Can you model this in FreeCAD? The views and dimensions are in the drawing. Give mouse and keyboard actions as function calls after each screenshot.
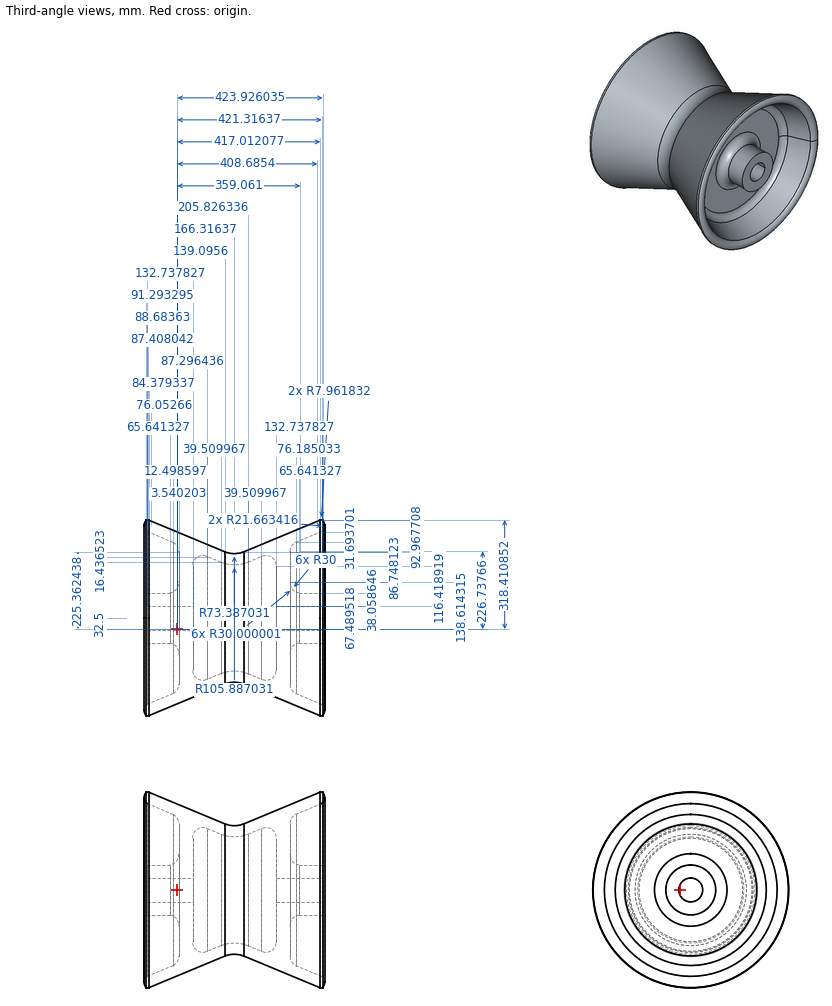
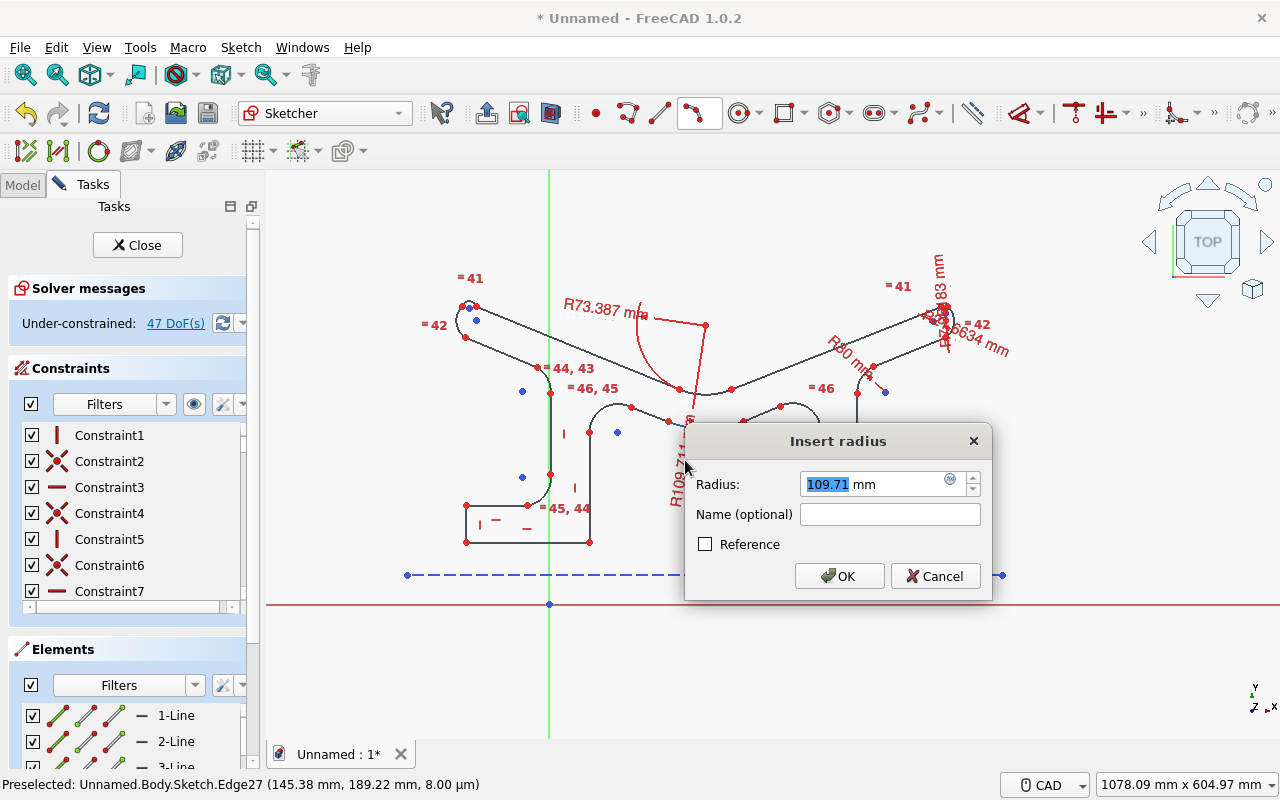
text(105.887031)
key(Return)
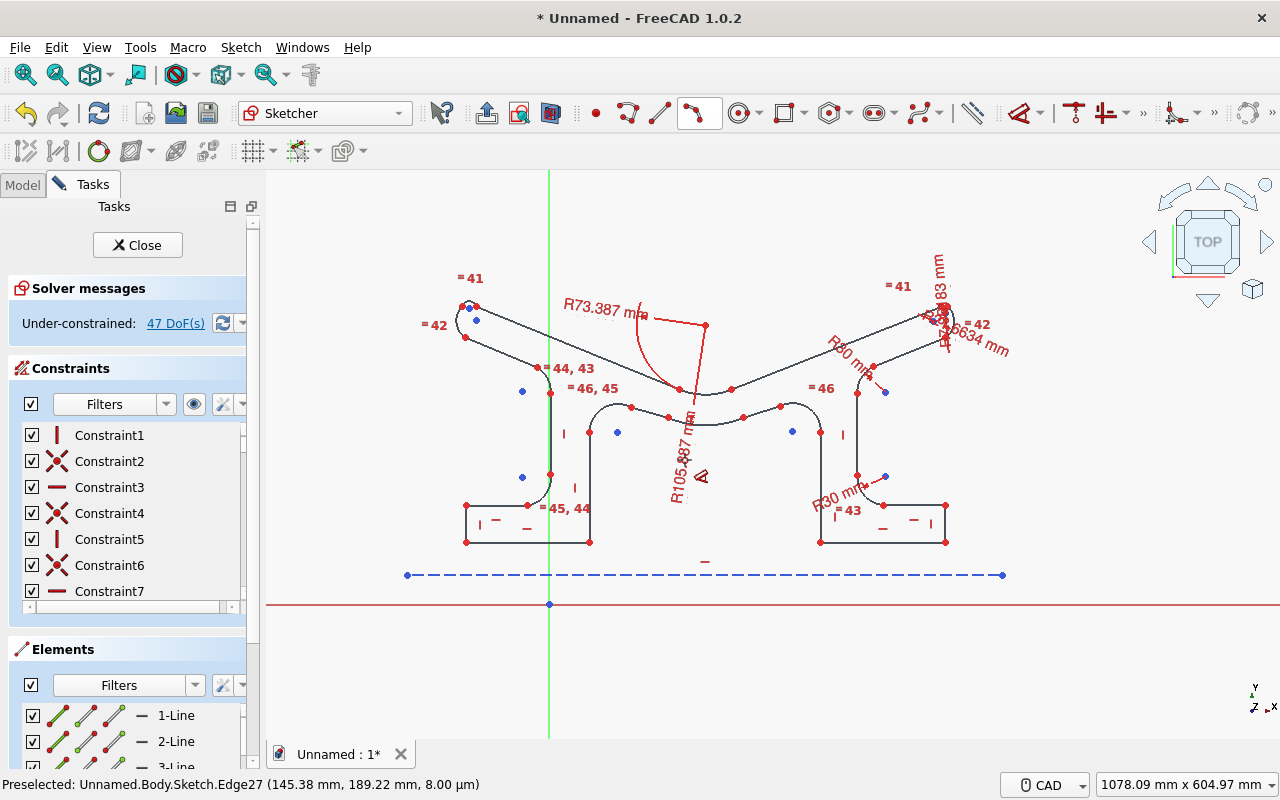
scroll(408, 575, up, 2)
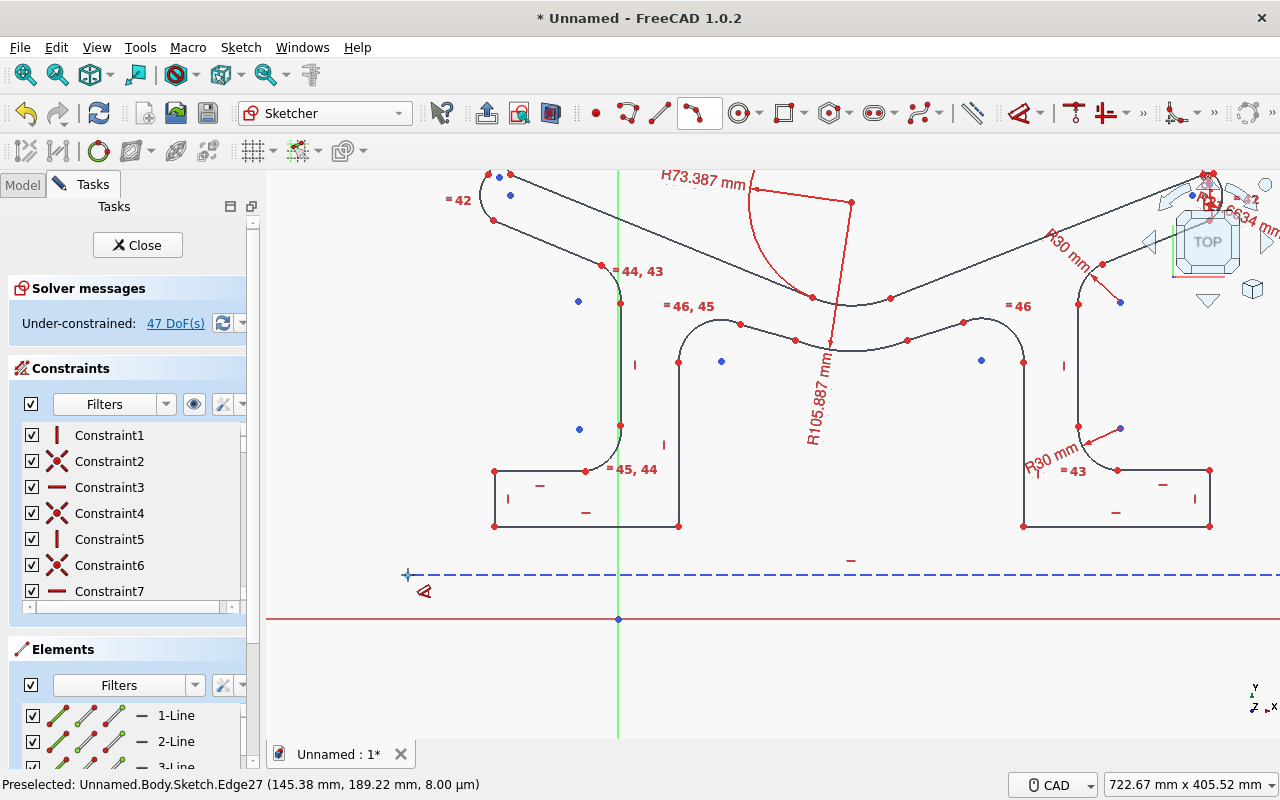
click(408, 575)
click(374, 597)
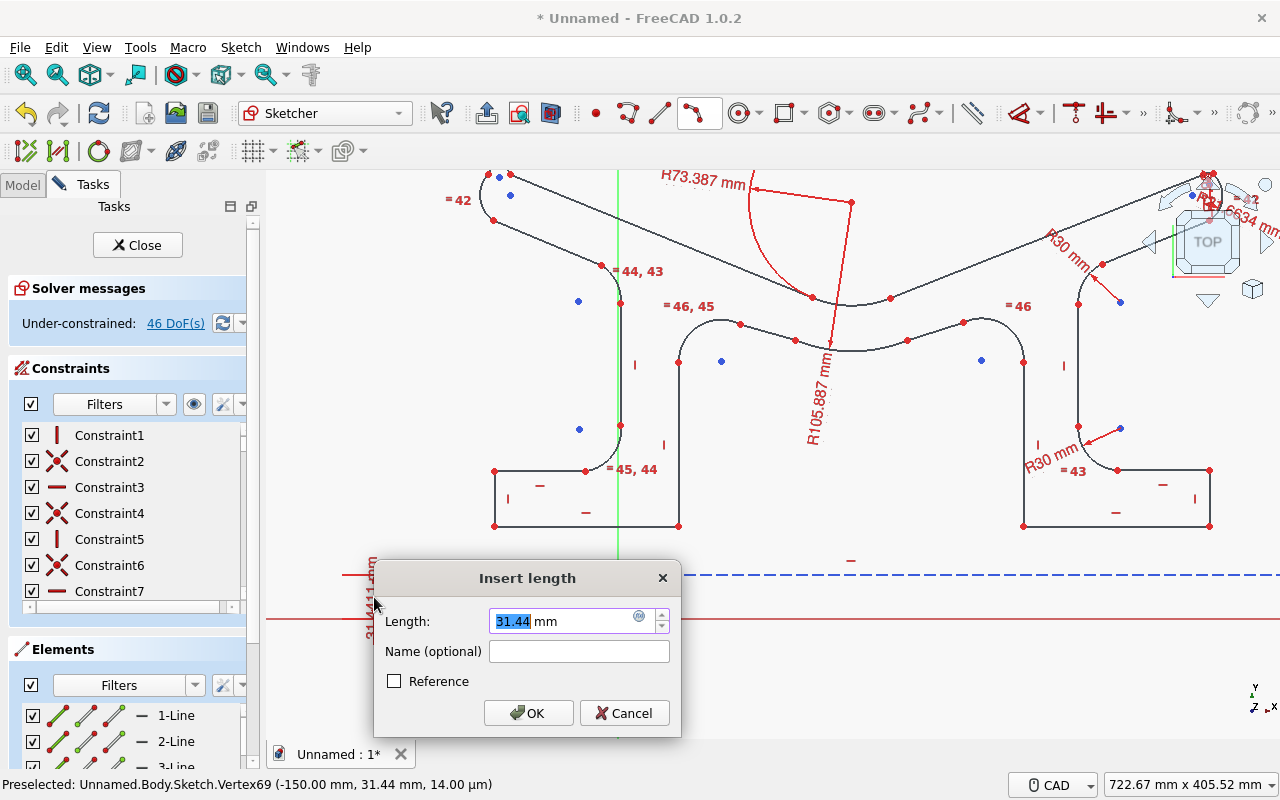
text(32.5)
key(Return)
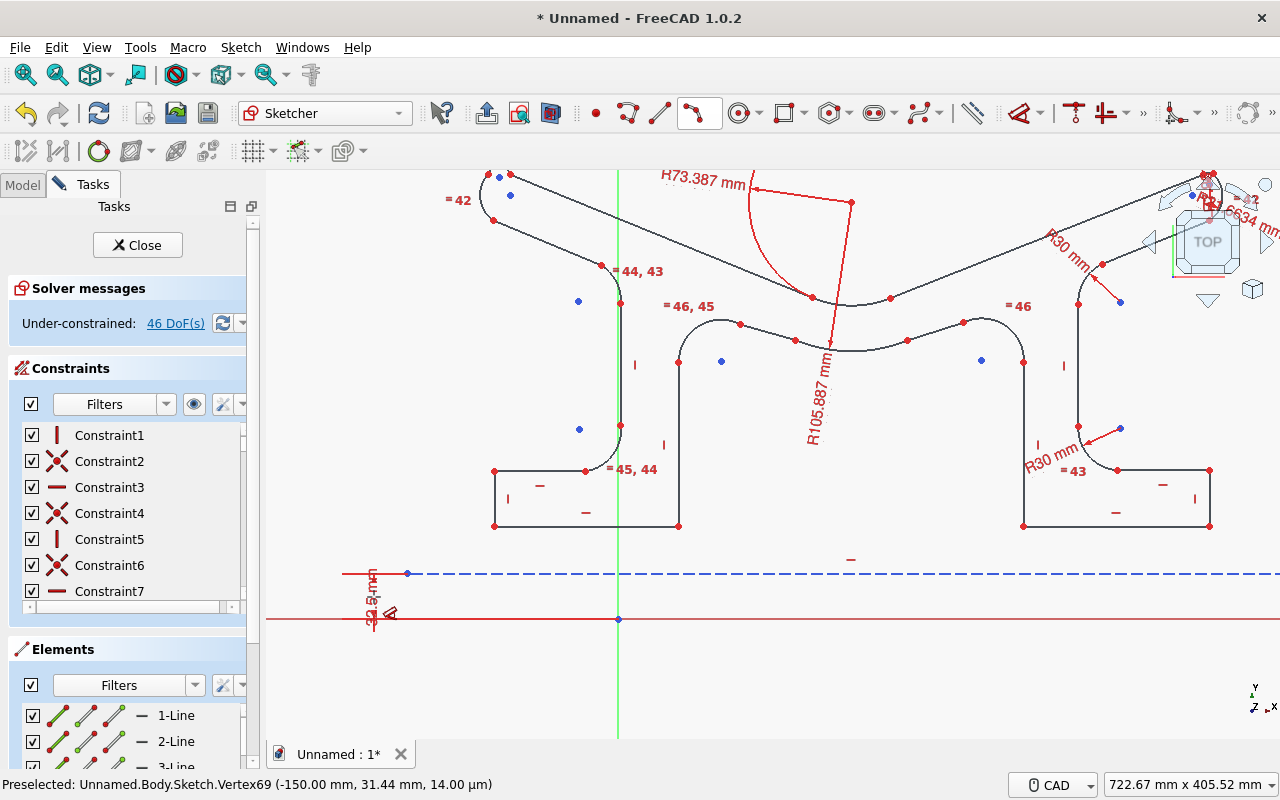
scroll(405, 575, down, 2)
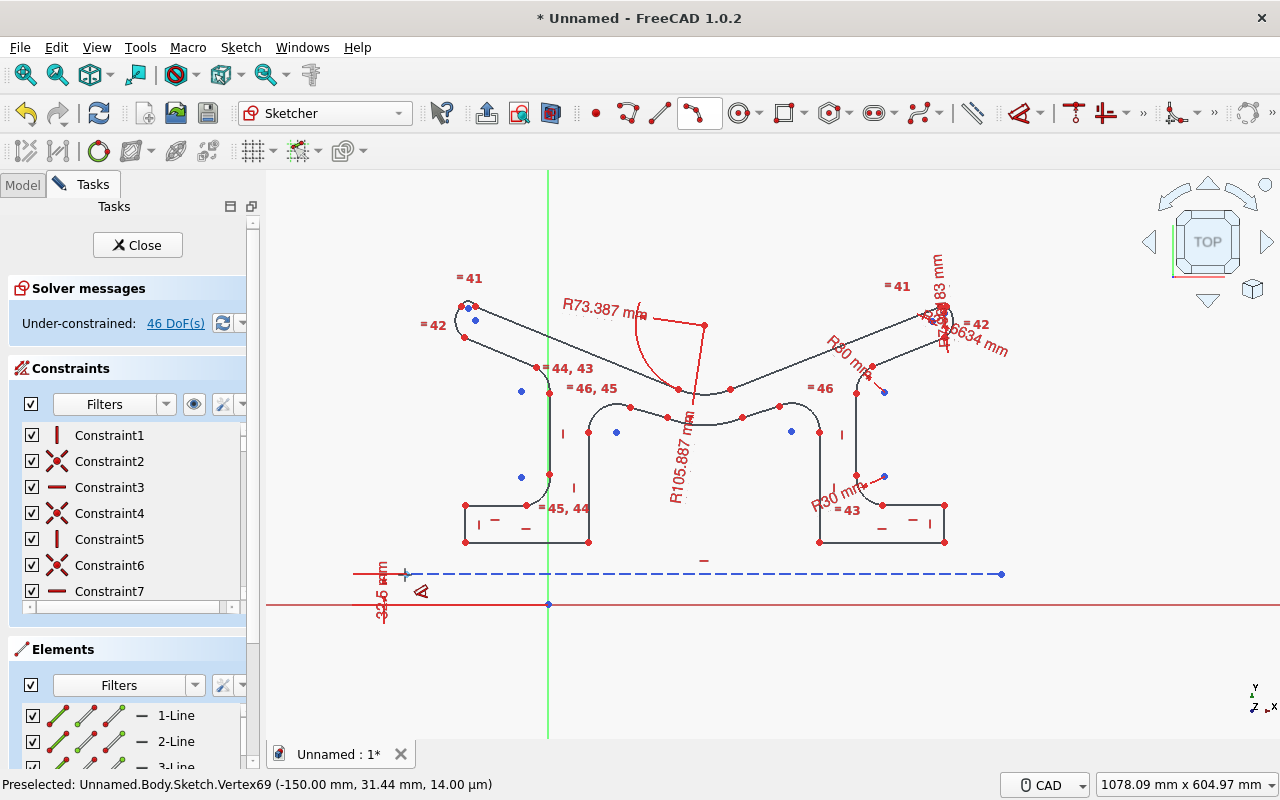
click(885, 392)
click(716, 639)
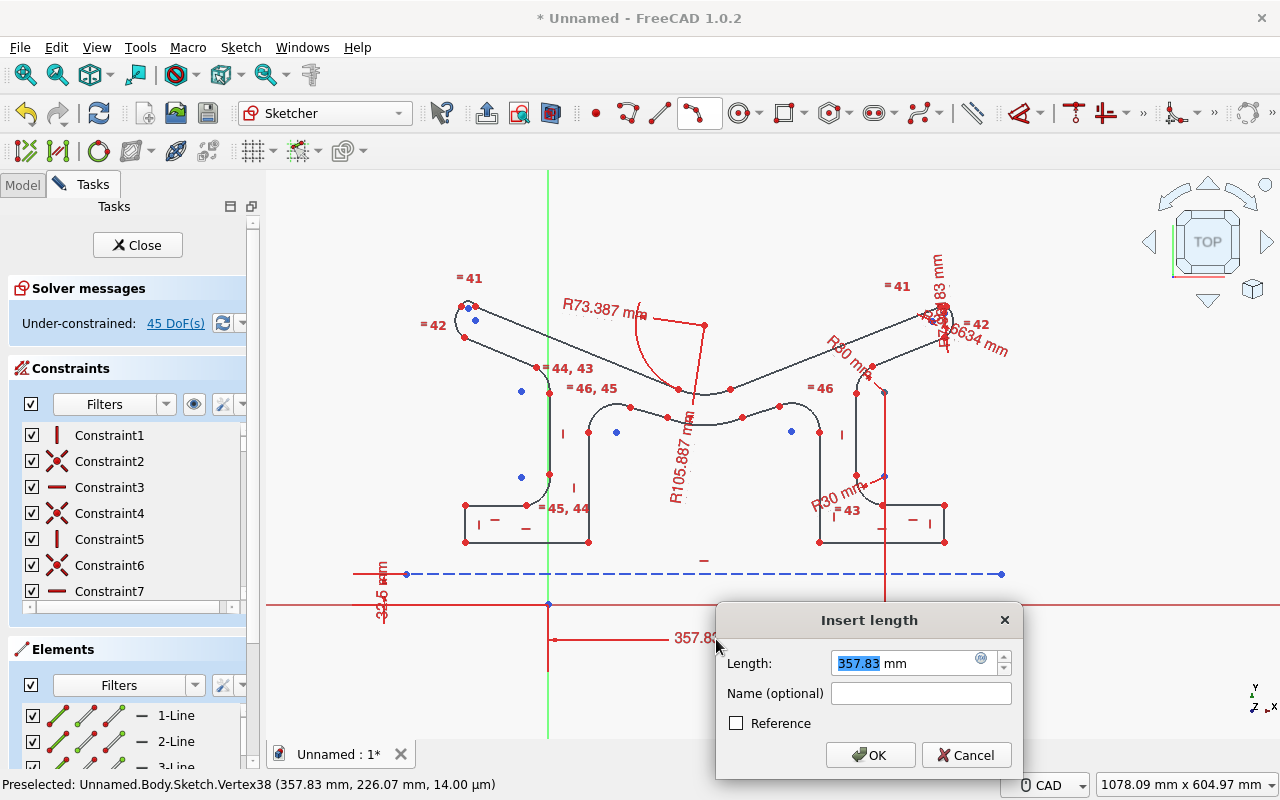
text(359.061)
key(Return)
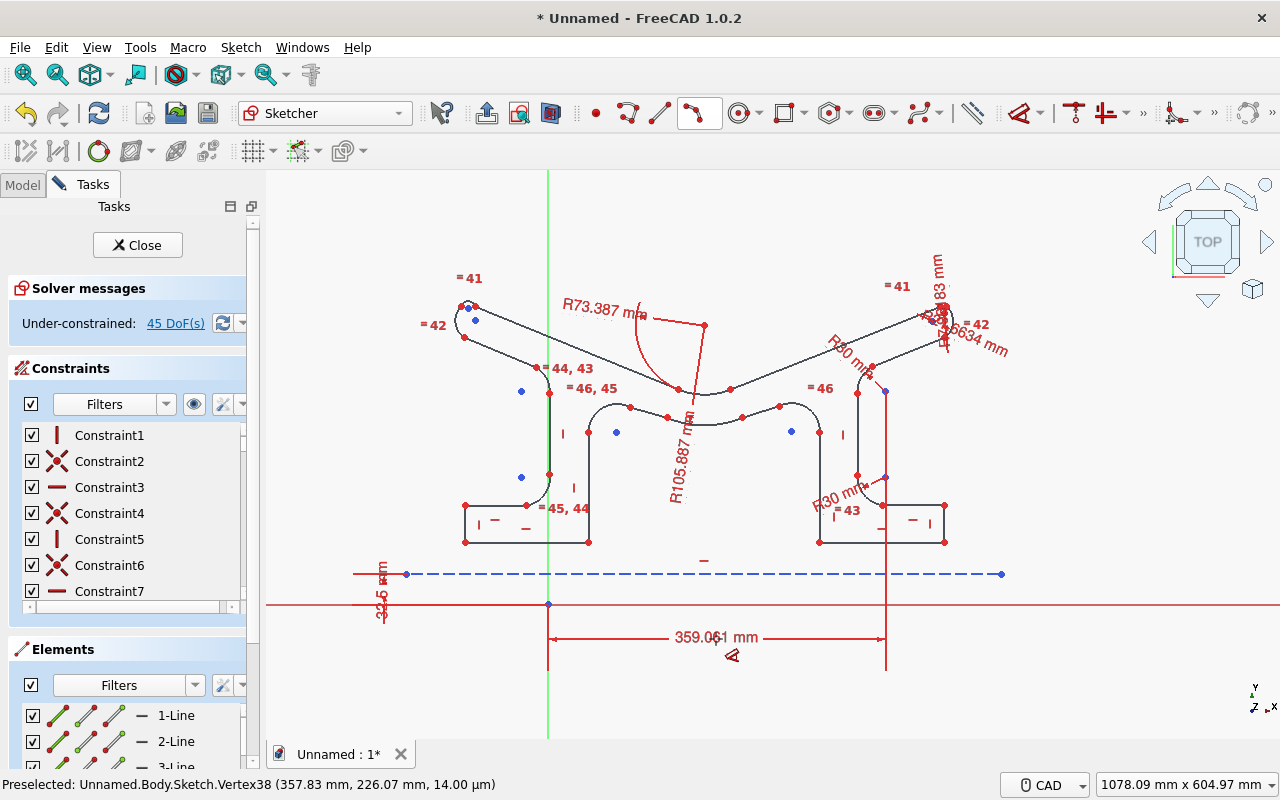
click(944, 532)
click(978, 524)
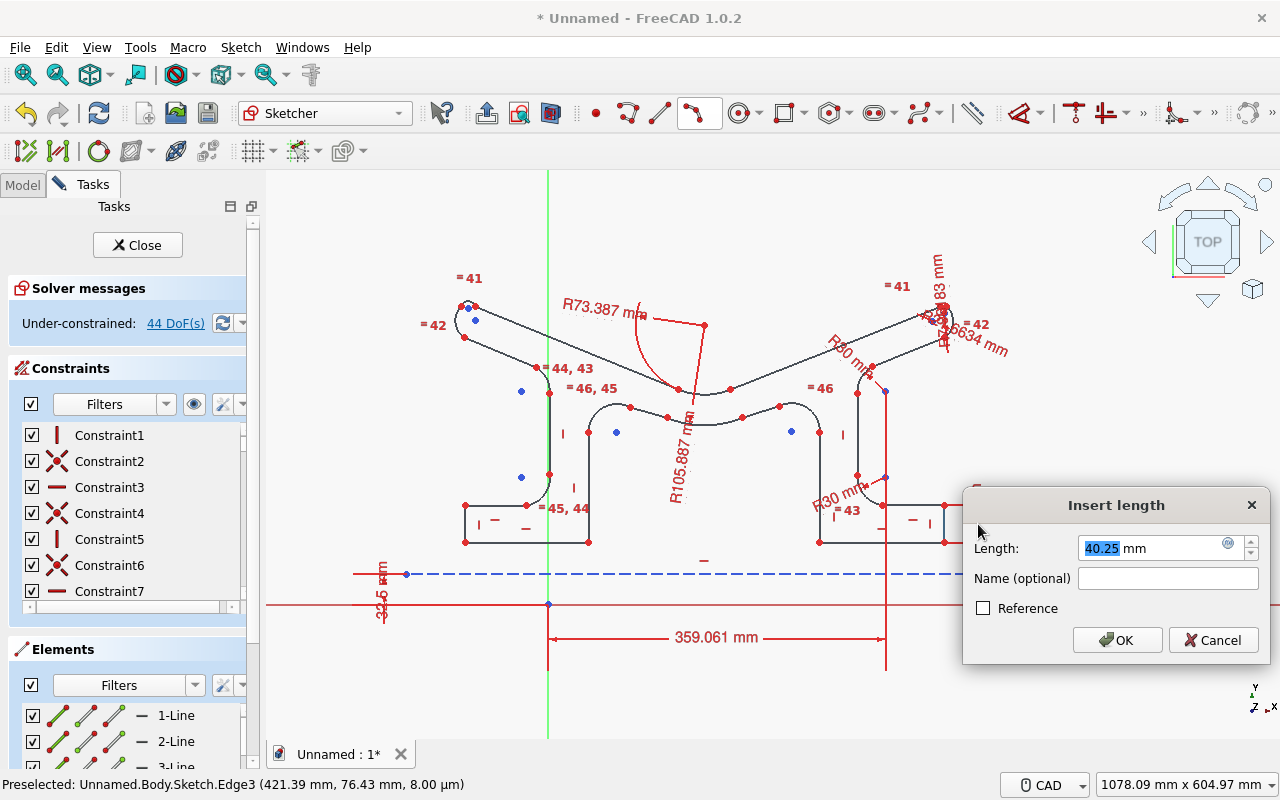
text(38.058646)
key(Return)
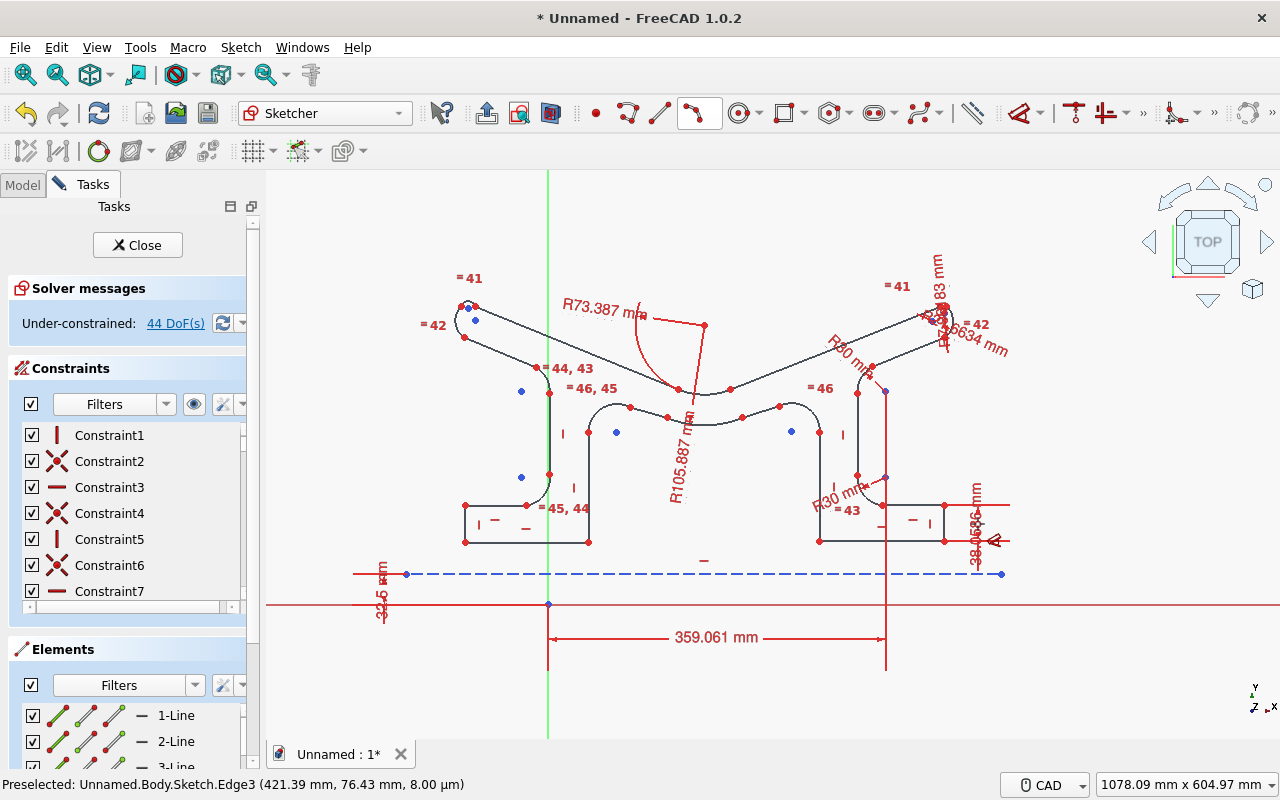
click(926, 505)
click(913, 471)